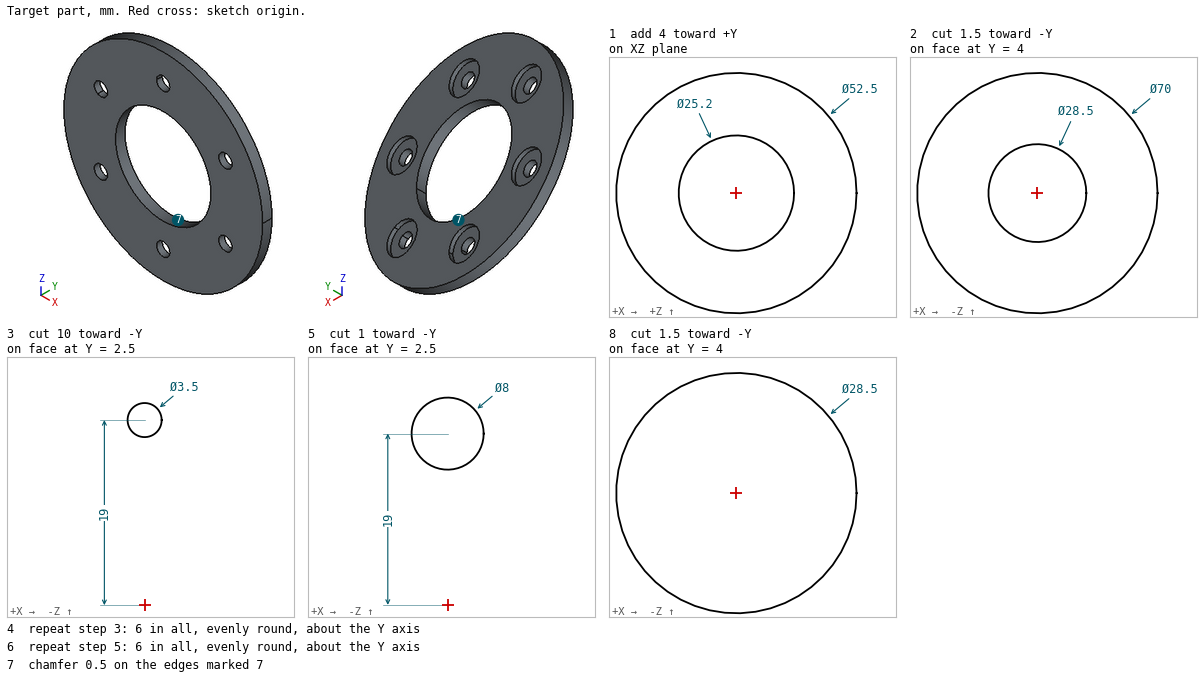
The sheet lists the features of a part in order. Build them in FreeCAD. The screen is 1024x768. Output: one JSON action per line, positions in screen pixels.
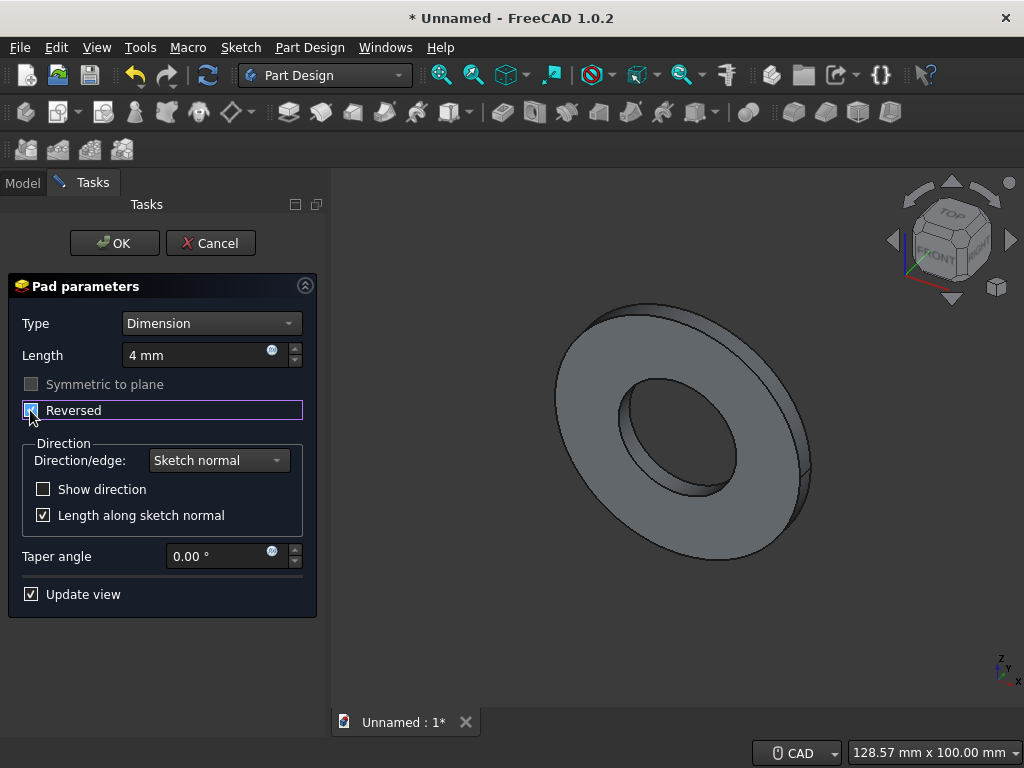
{"action": "left_click", "coordinate": [115, 243]}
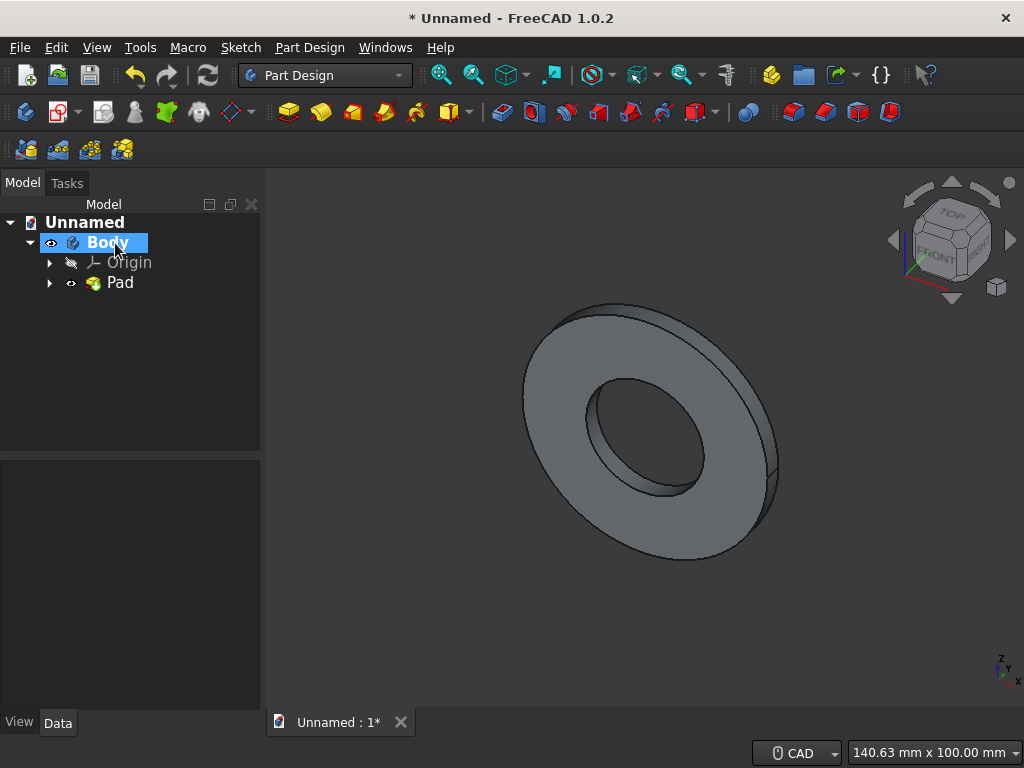
{"action": "key", "text": "4"}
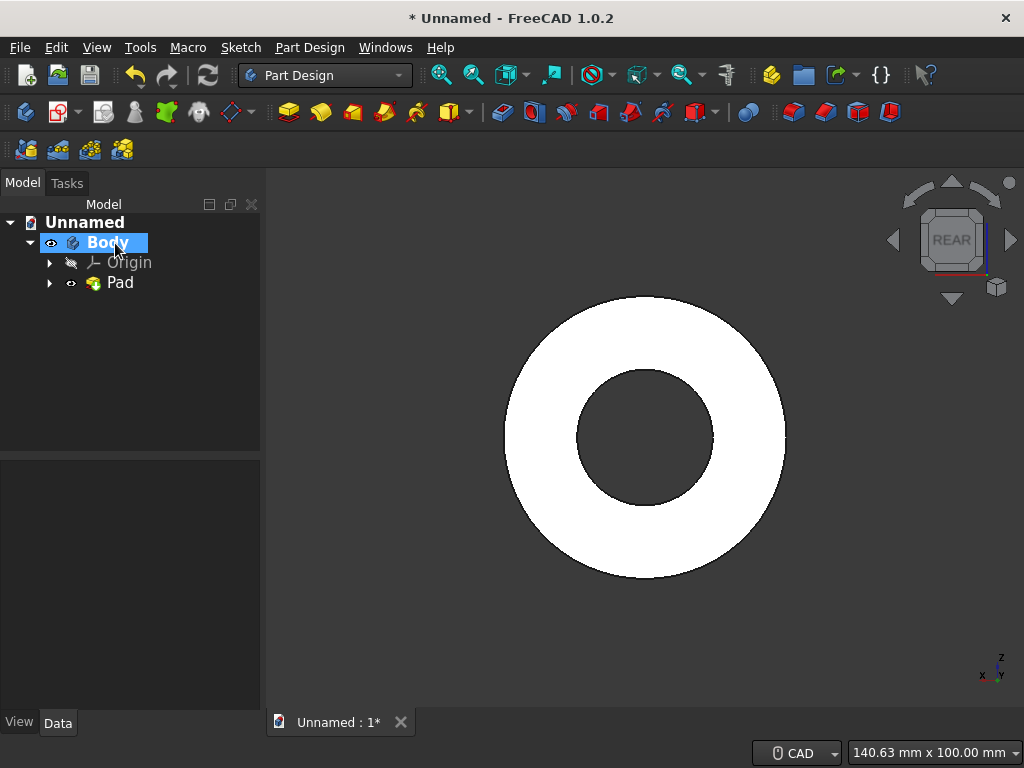
{"action": "left_click", "coordinate": [564, 356]}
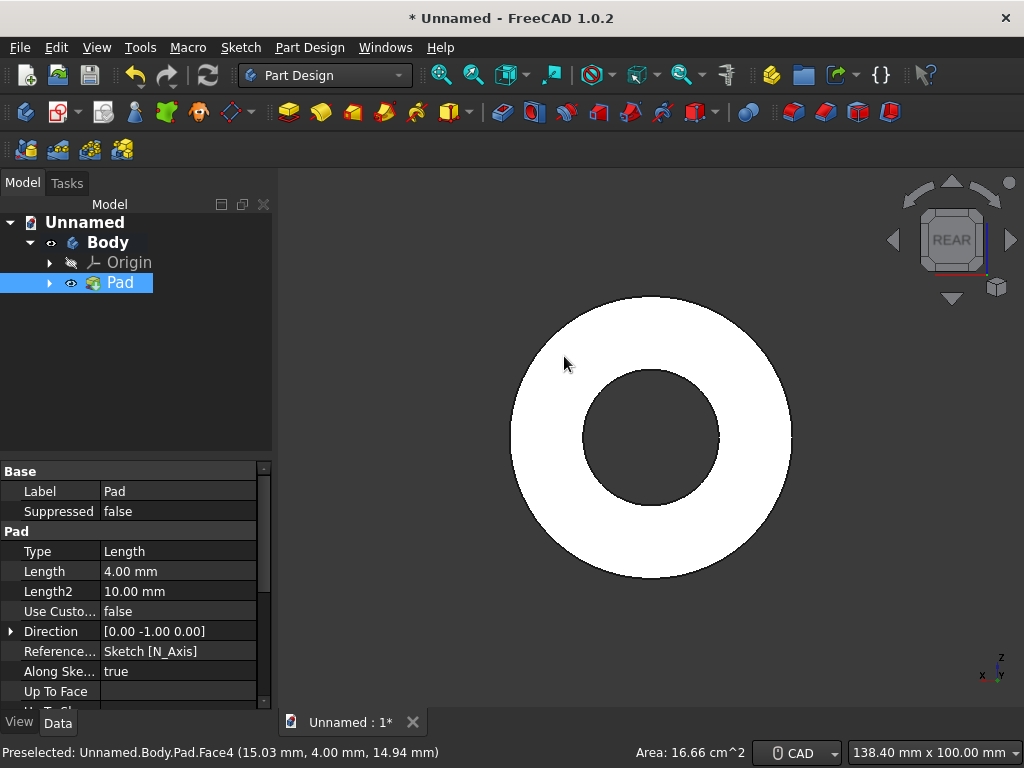
{"action": "left_click", "coordinate": [58, 112]}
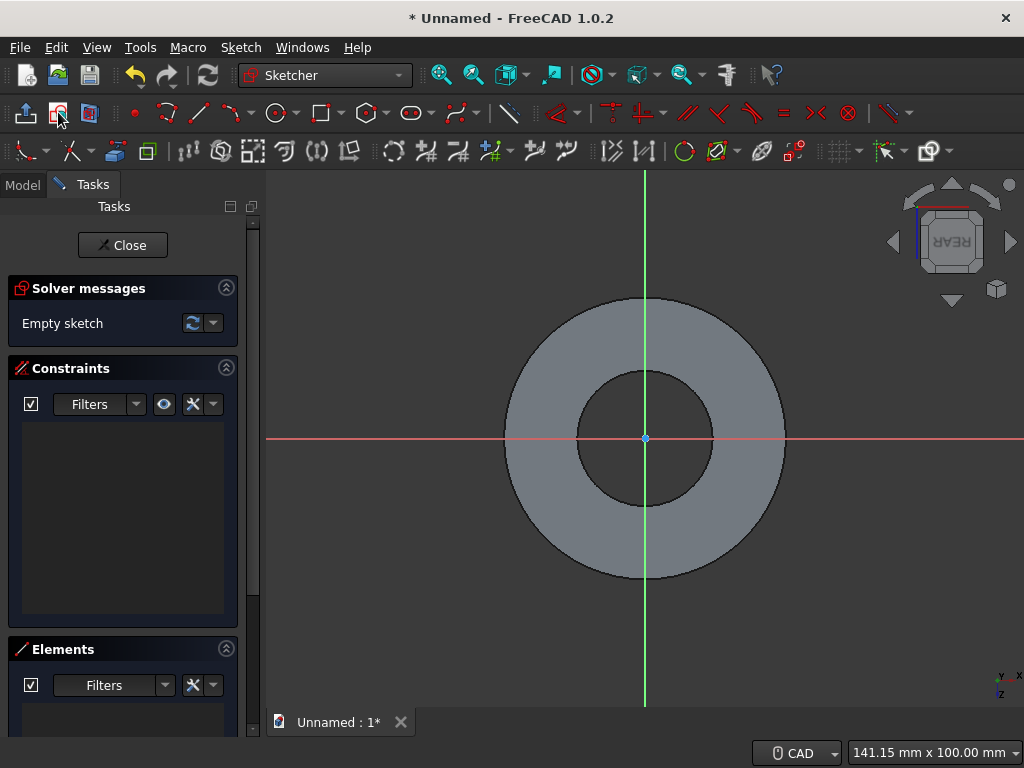
{"action": "left_click", "coordinate": [276, 114]}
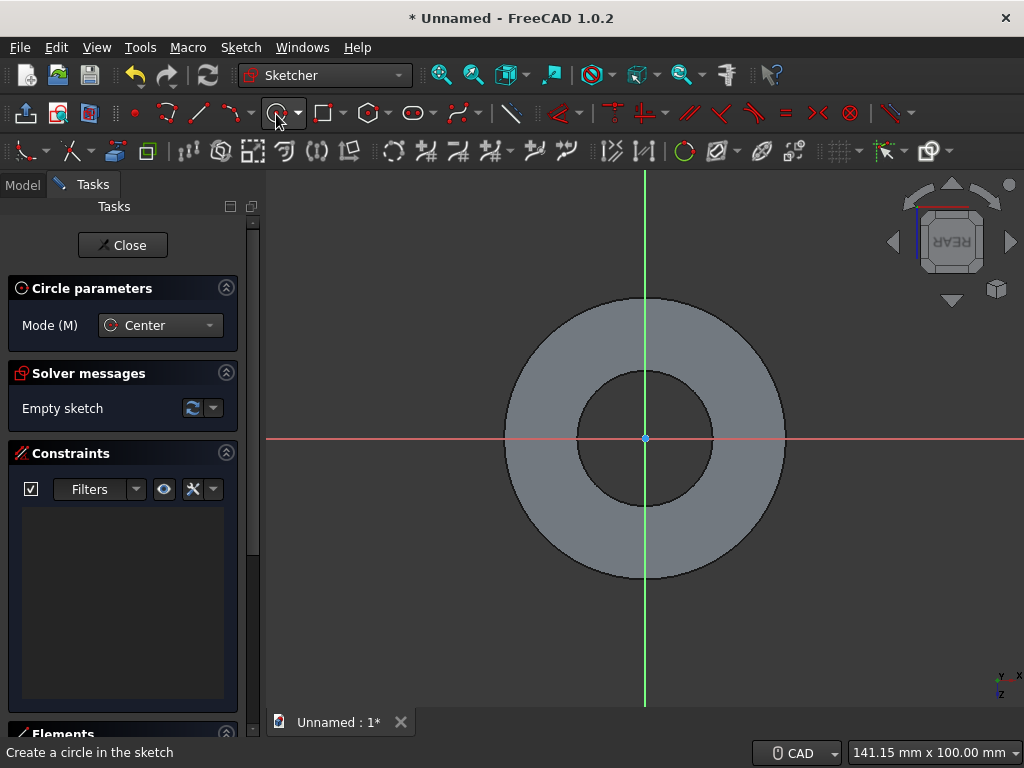
{"action": "left_click", "coordinate": [645, 439]}
{"action": "mouse_move", "coordinate": [778, 306]}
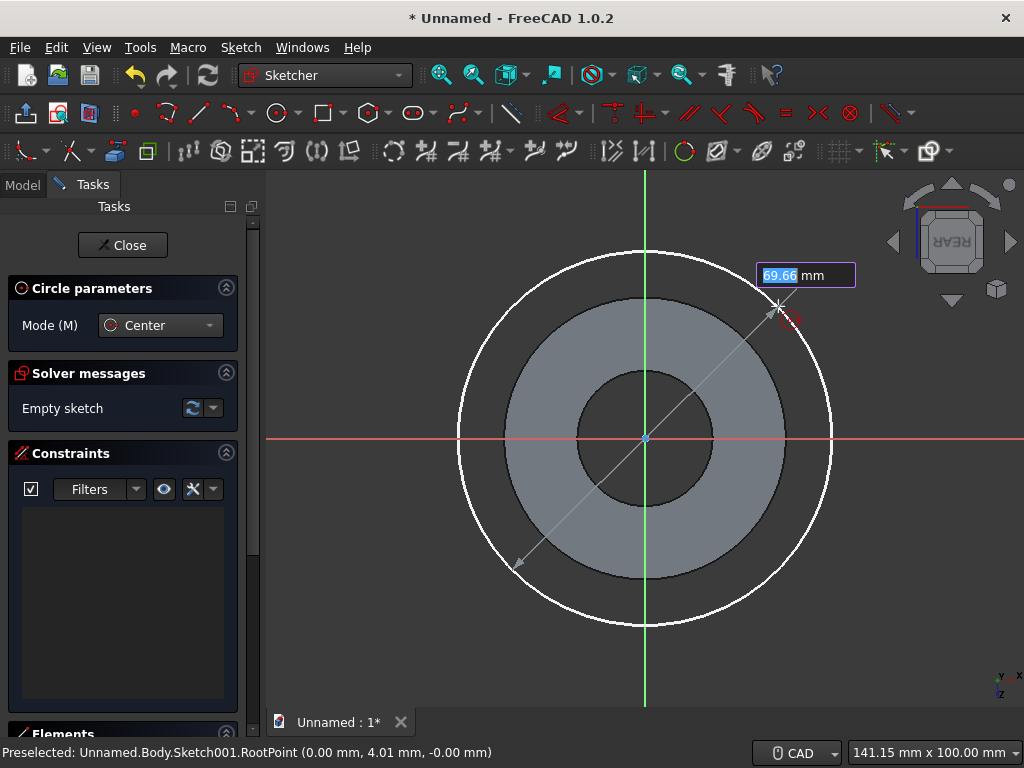
{"action": "type", "text": "70"}
{"action": "key", "text": "Return"}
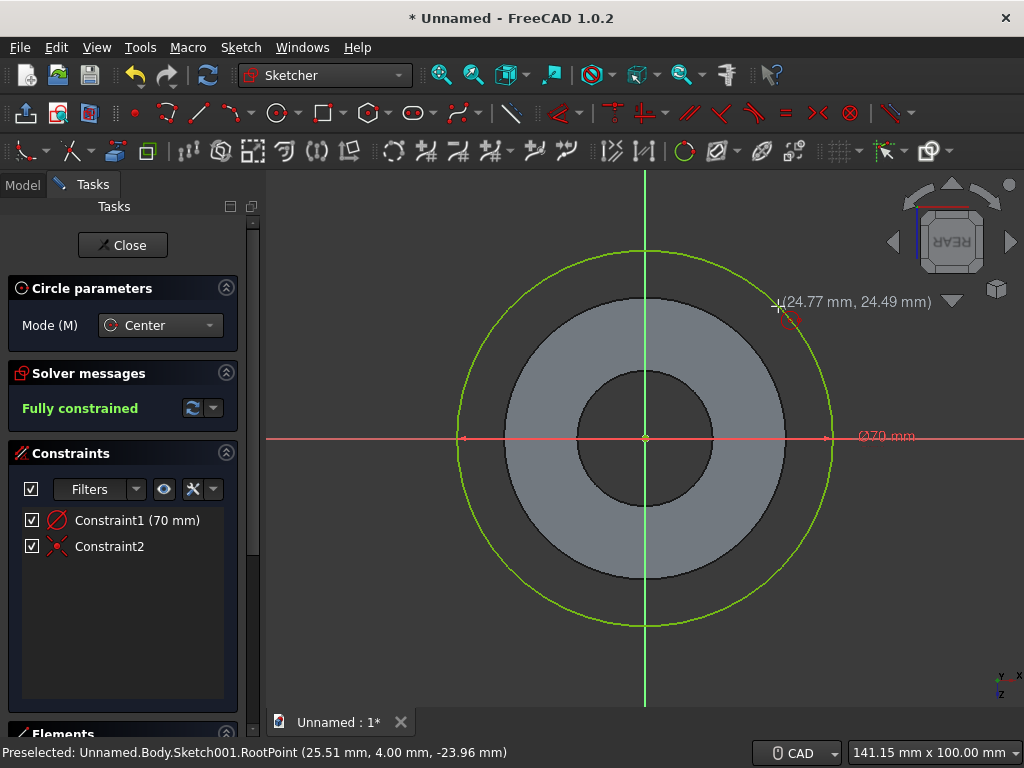
{"action": "left_click", "coordinate": [645, 439]}
{"action": "mouse_move", "coordinate": [699, 384]}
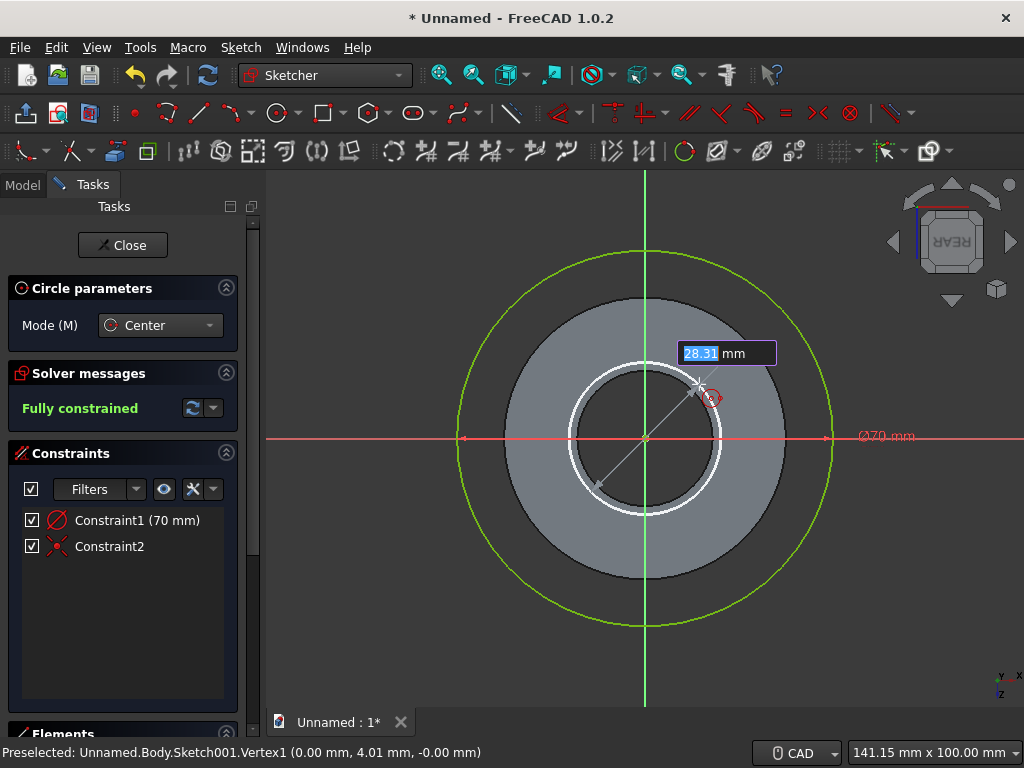
{"action": "type", "text": "28.5"}
{"action": "key", "text": "Return"}
{"action": "key", "text": "Escape"}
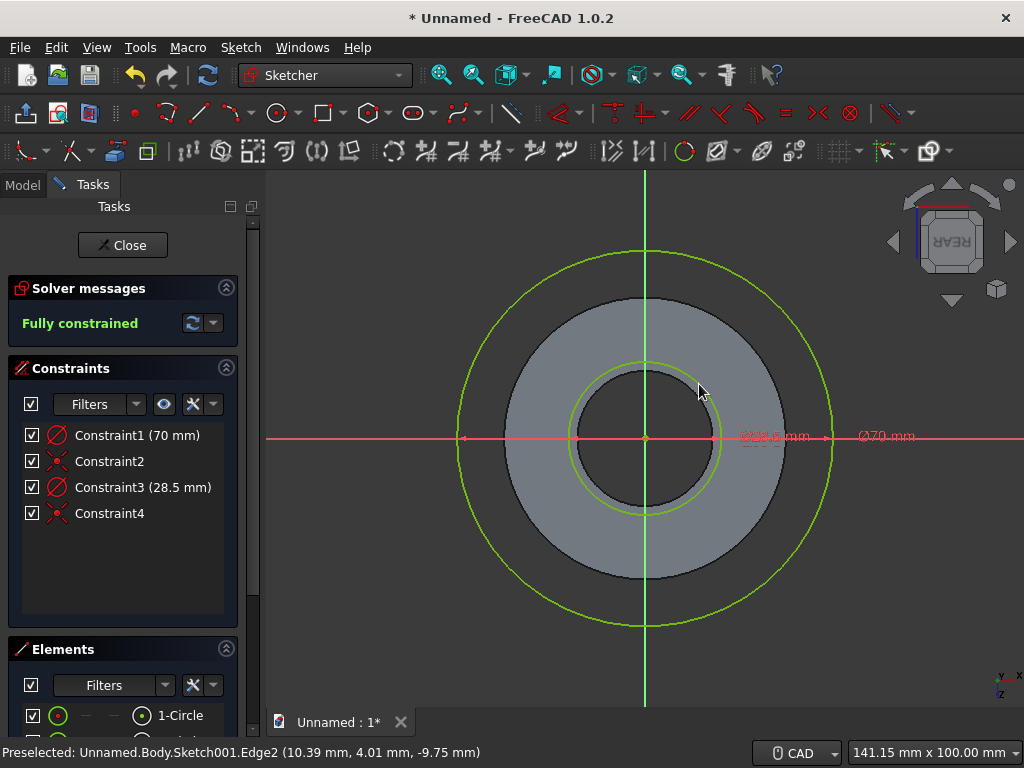
{"action": "left_click", "coordinate": [123, 245]}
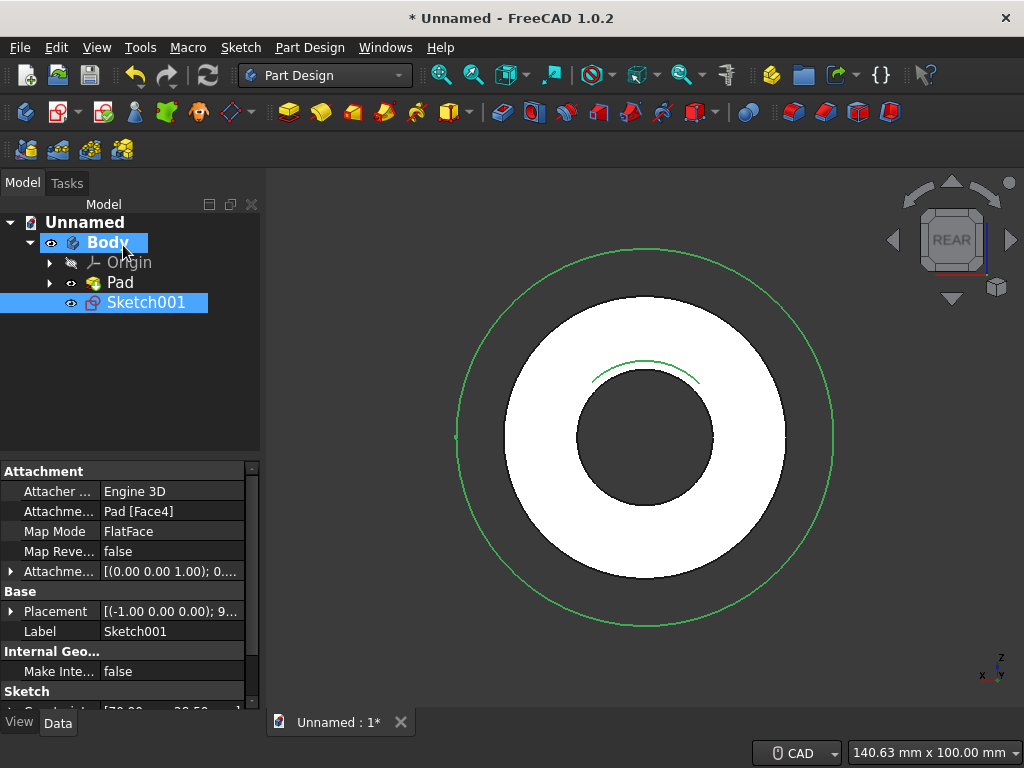
{"action": "left_click", "coordinate": [504, 112]}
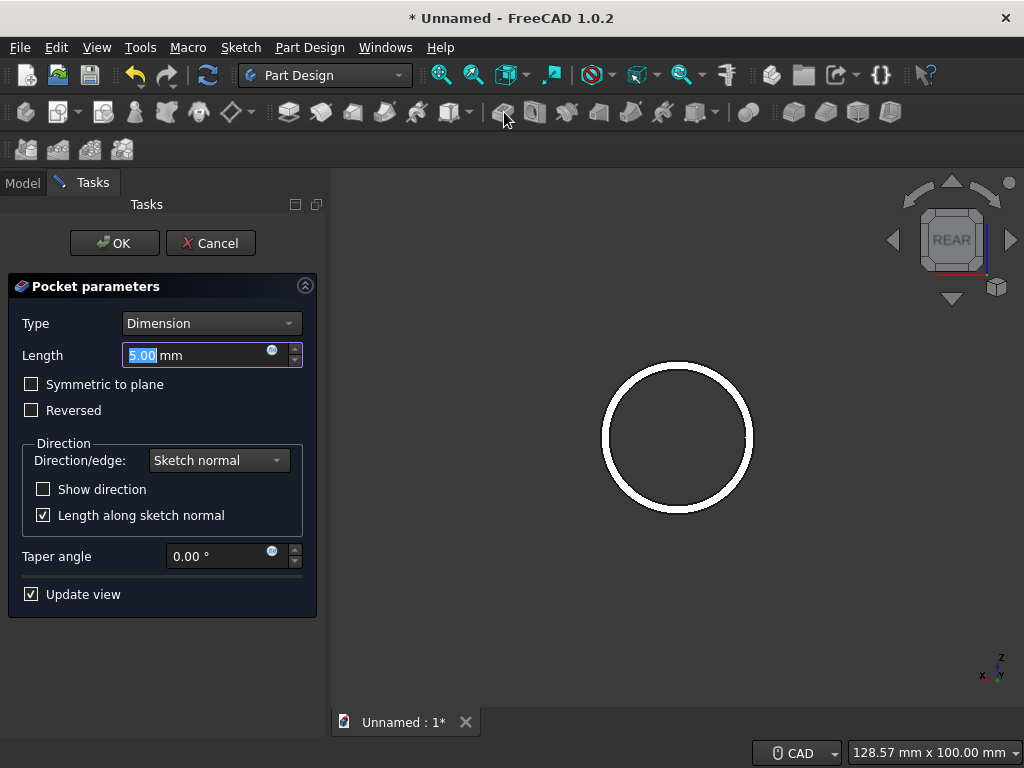
{"action": "type", "text": "1.5"}
{"action": "key", "text": "Tab"}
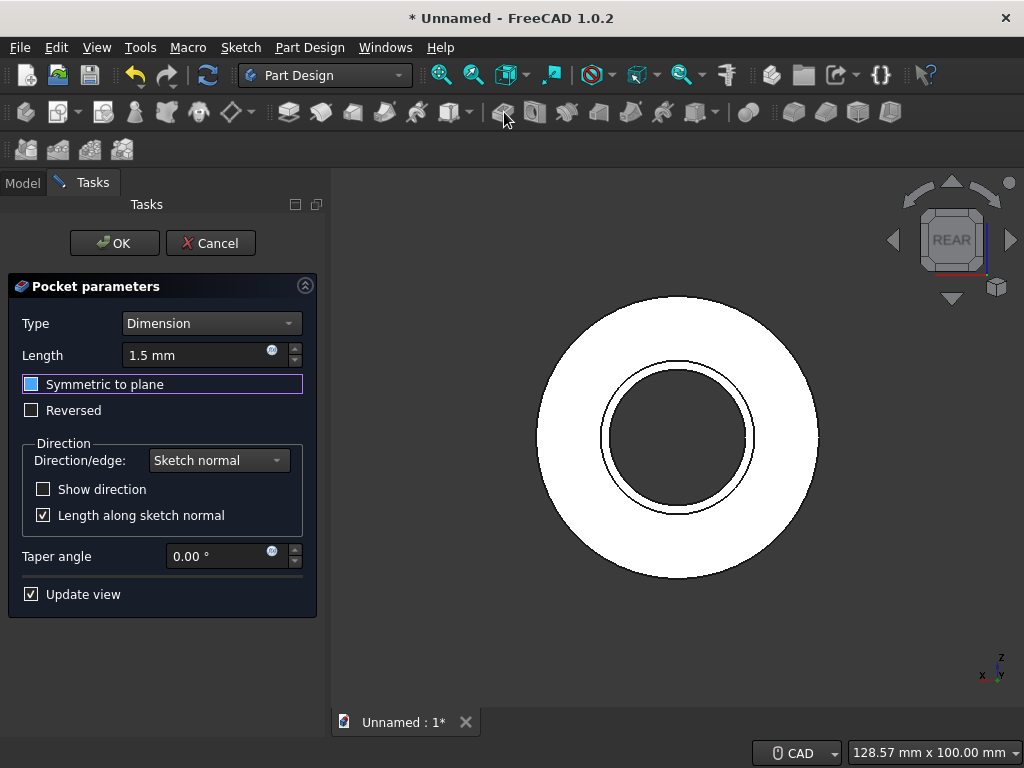
{"action": "left_click", "coordinate": [115, 243]}